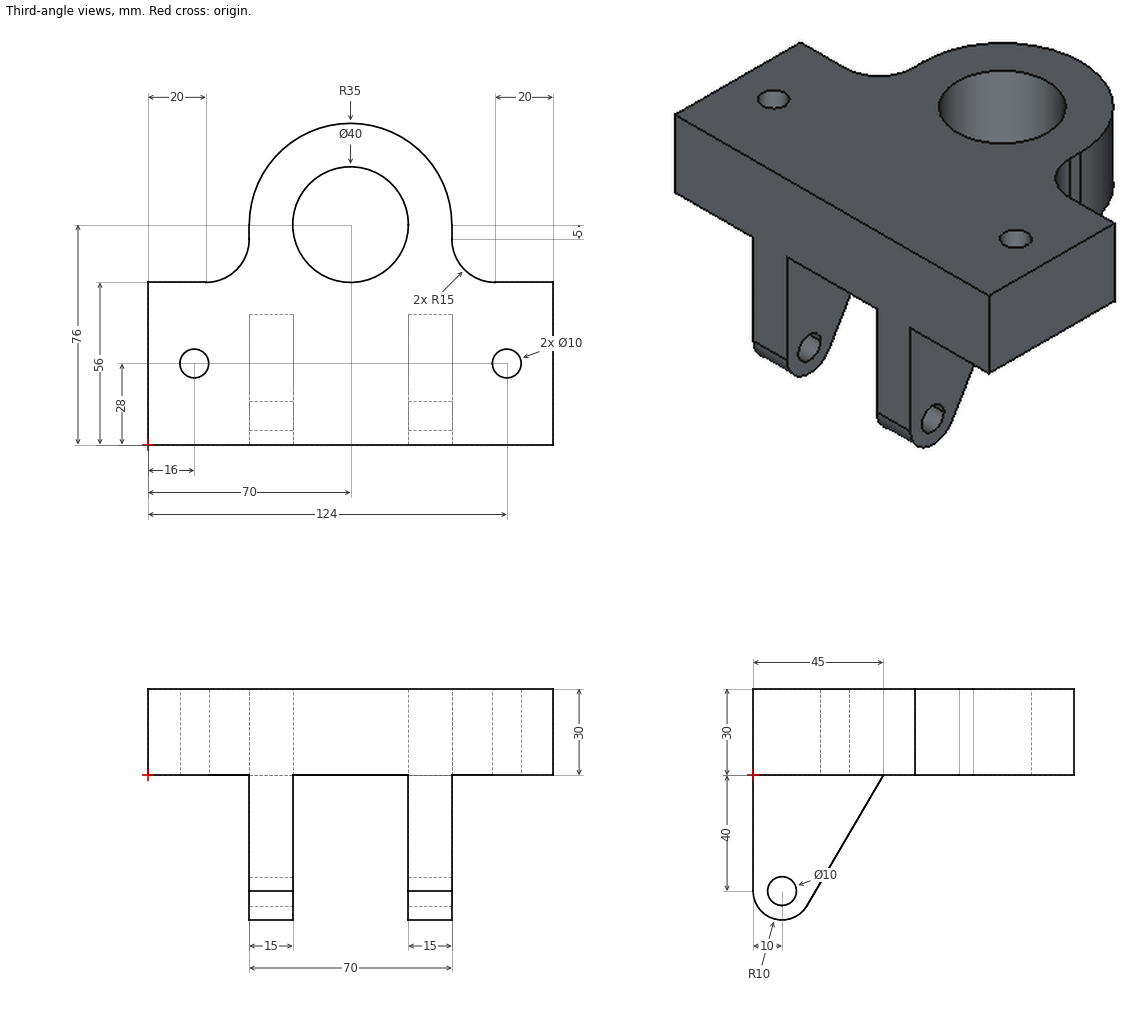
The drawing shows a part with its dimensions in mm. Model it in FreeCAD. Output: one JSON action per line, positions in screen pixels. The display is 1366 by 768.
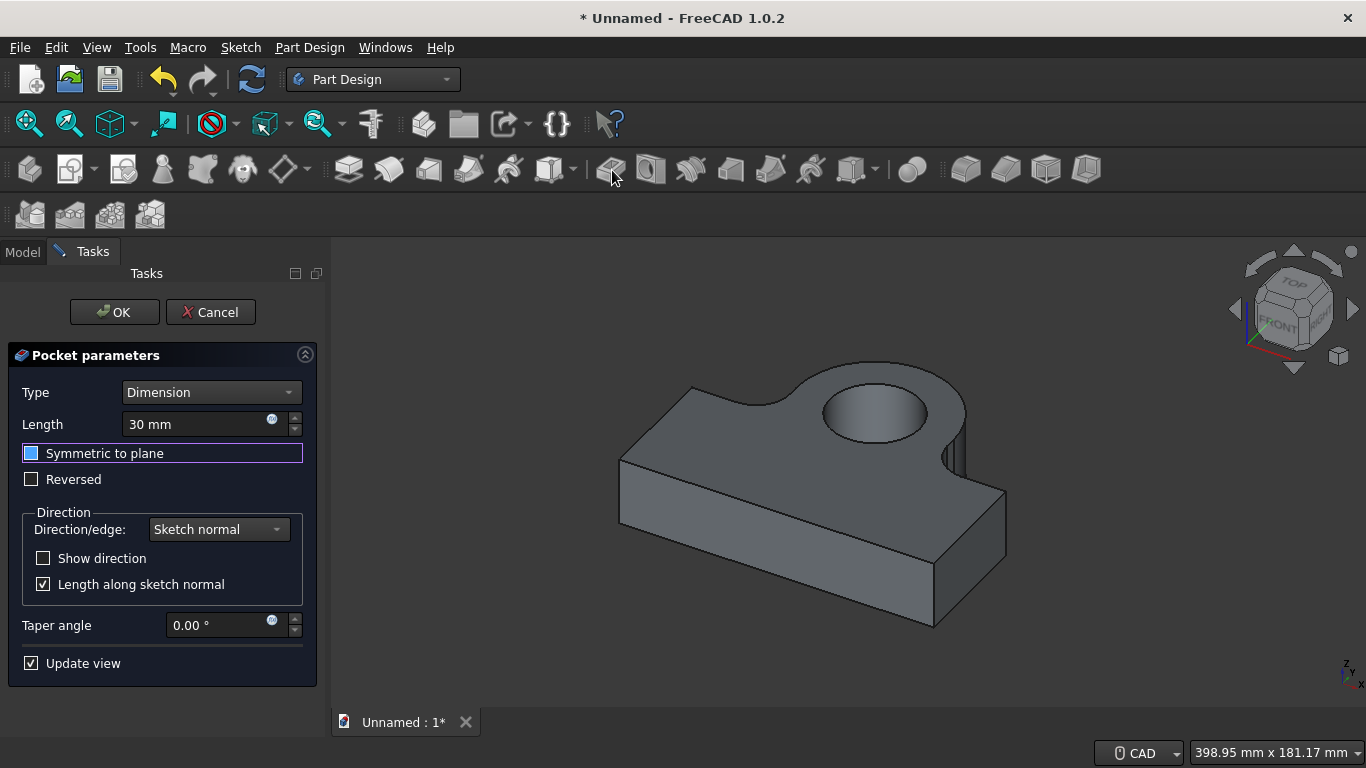
{"action": "left_click", "coordinate": [115, 312]}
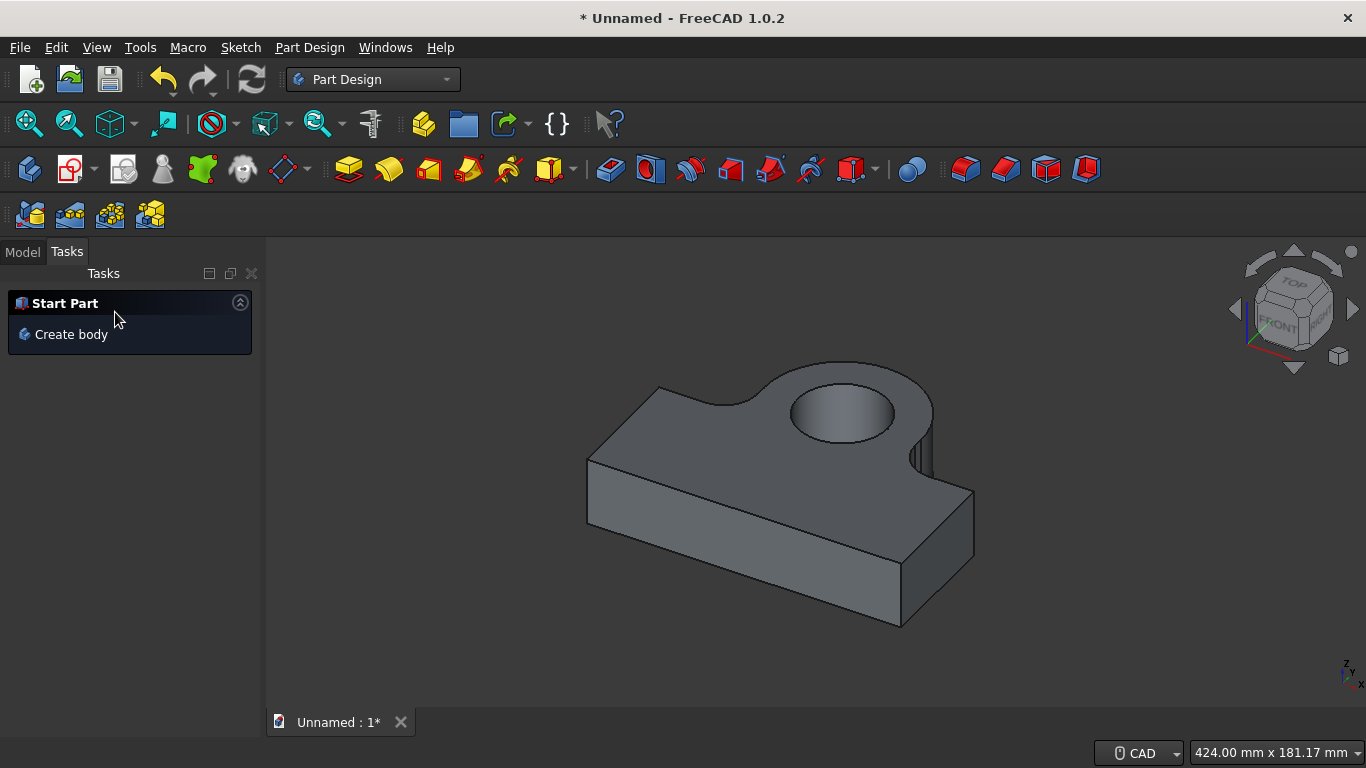
{"action": "key", "text": "6"}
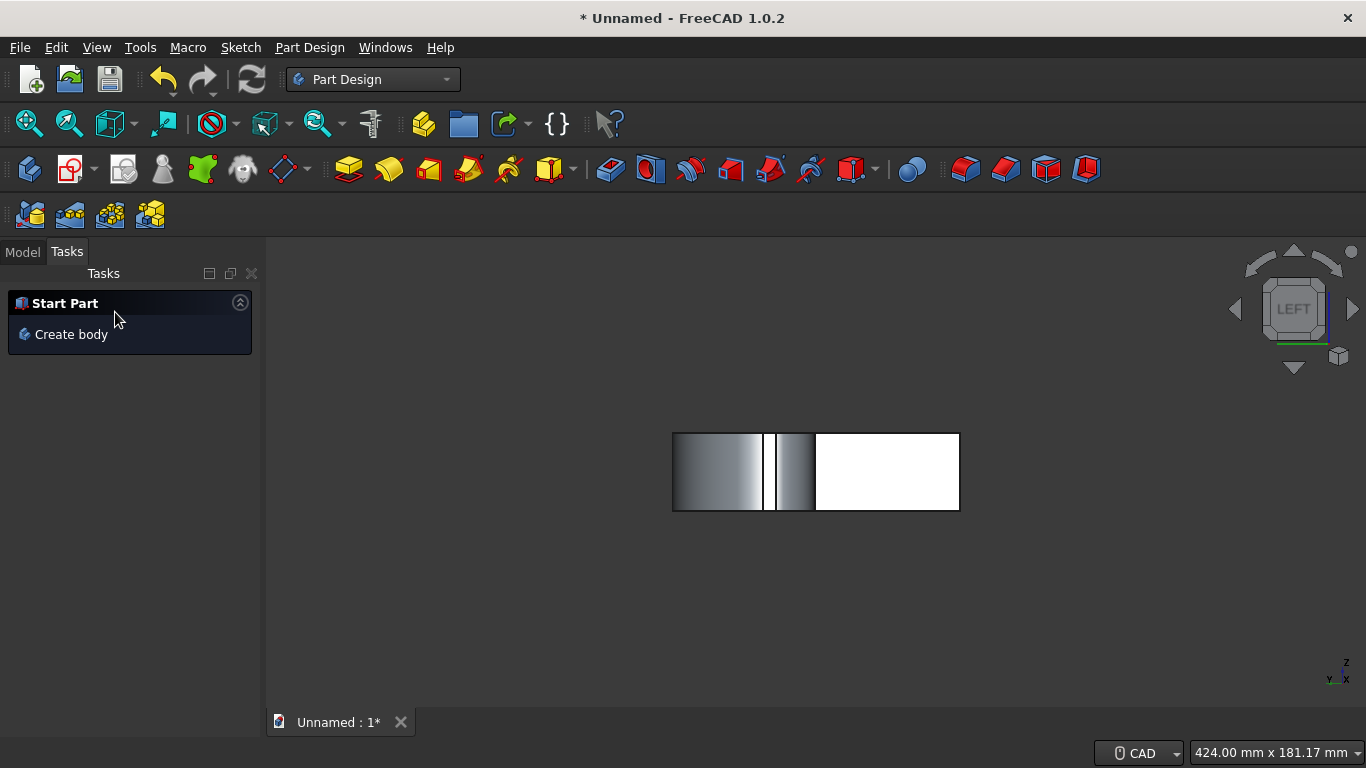
{"action": "left_click", "coordinate": [30, 124]}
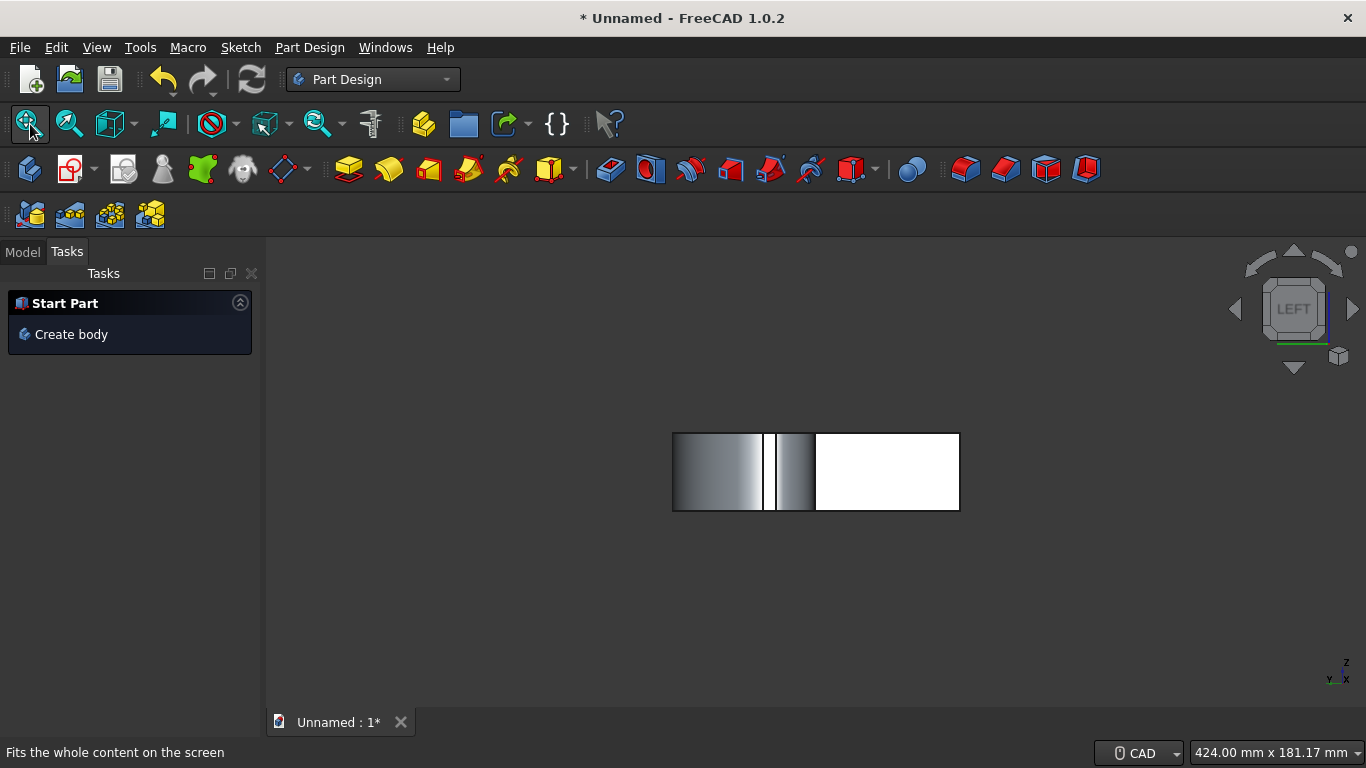
{"action": "scroll", "coordinate": [769, 449], "scroll_direction": "up", "scroll_amount": 4}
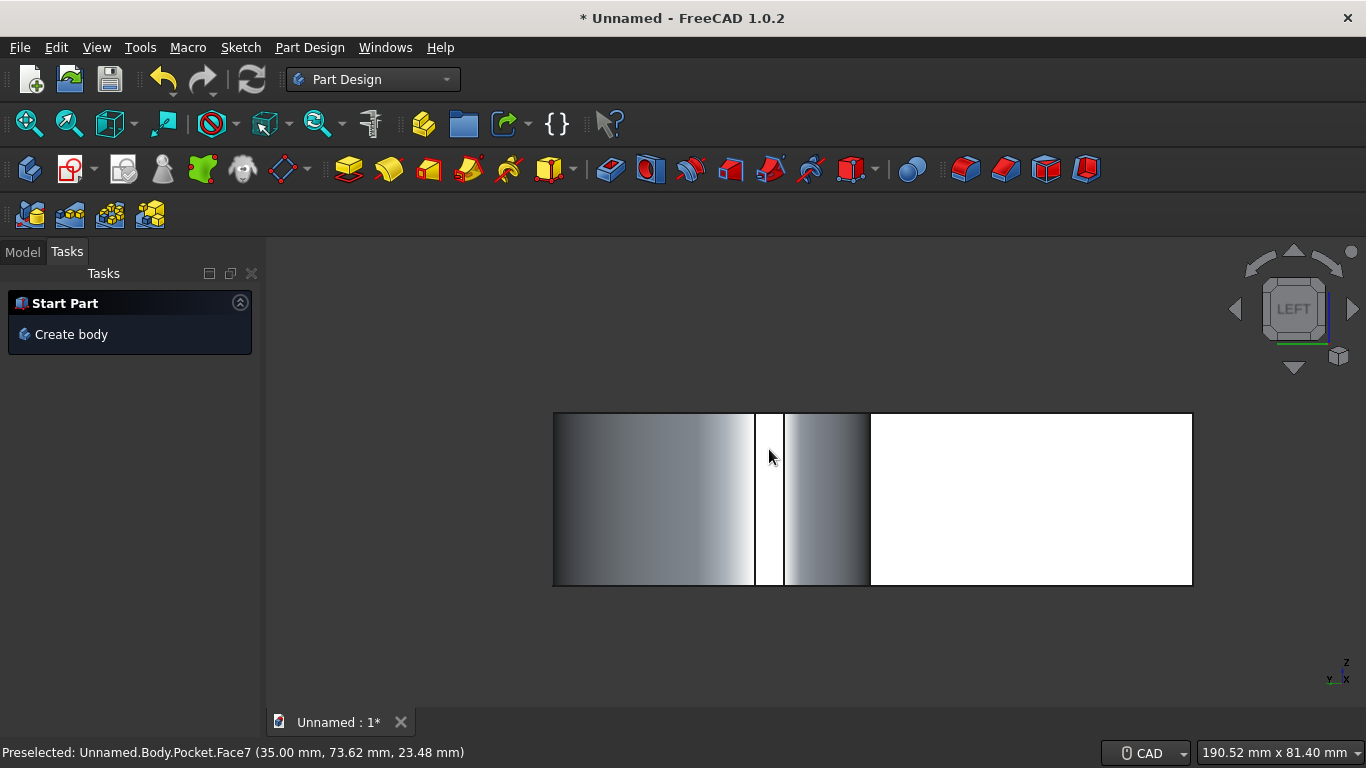
{"action": "left_click", "coordinate": [769, 449]}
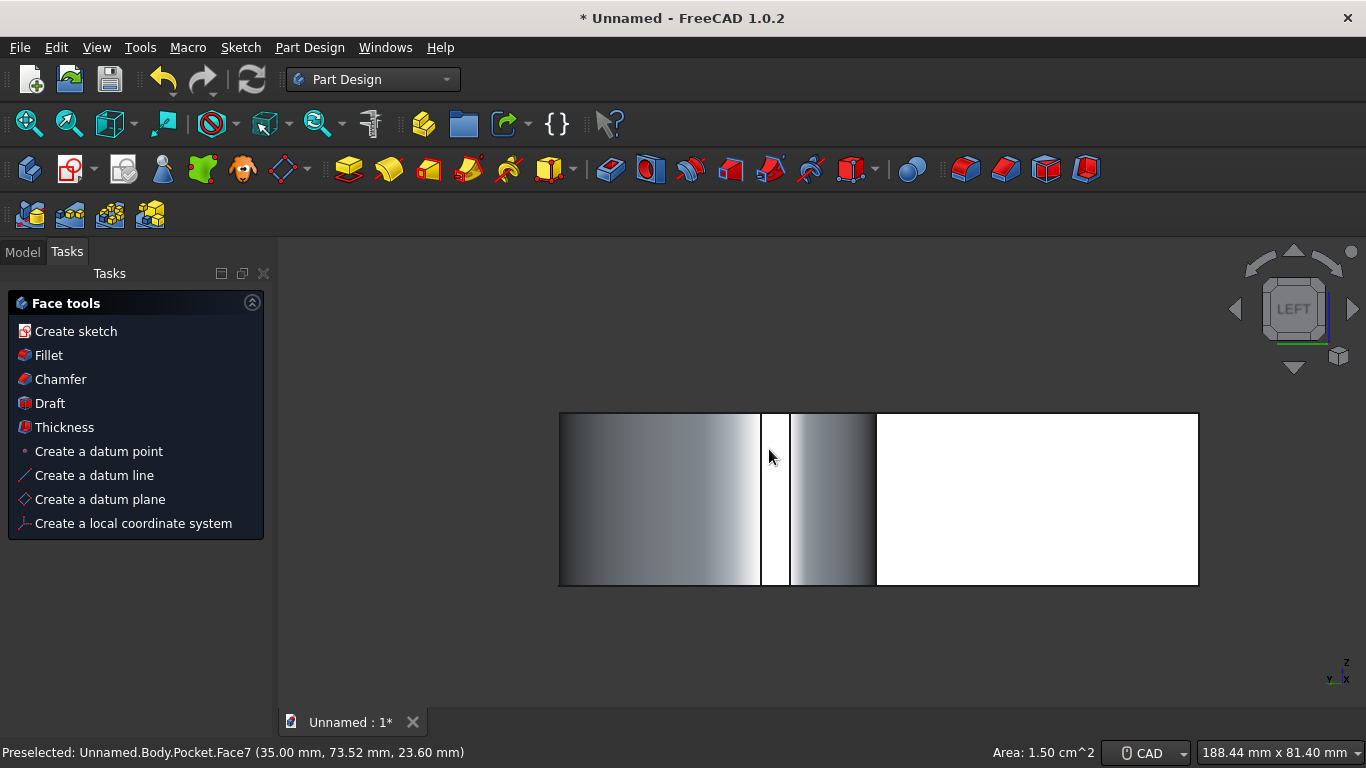
{"action": "left_click", "coordinate": [70, 170]}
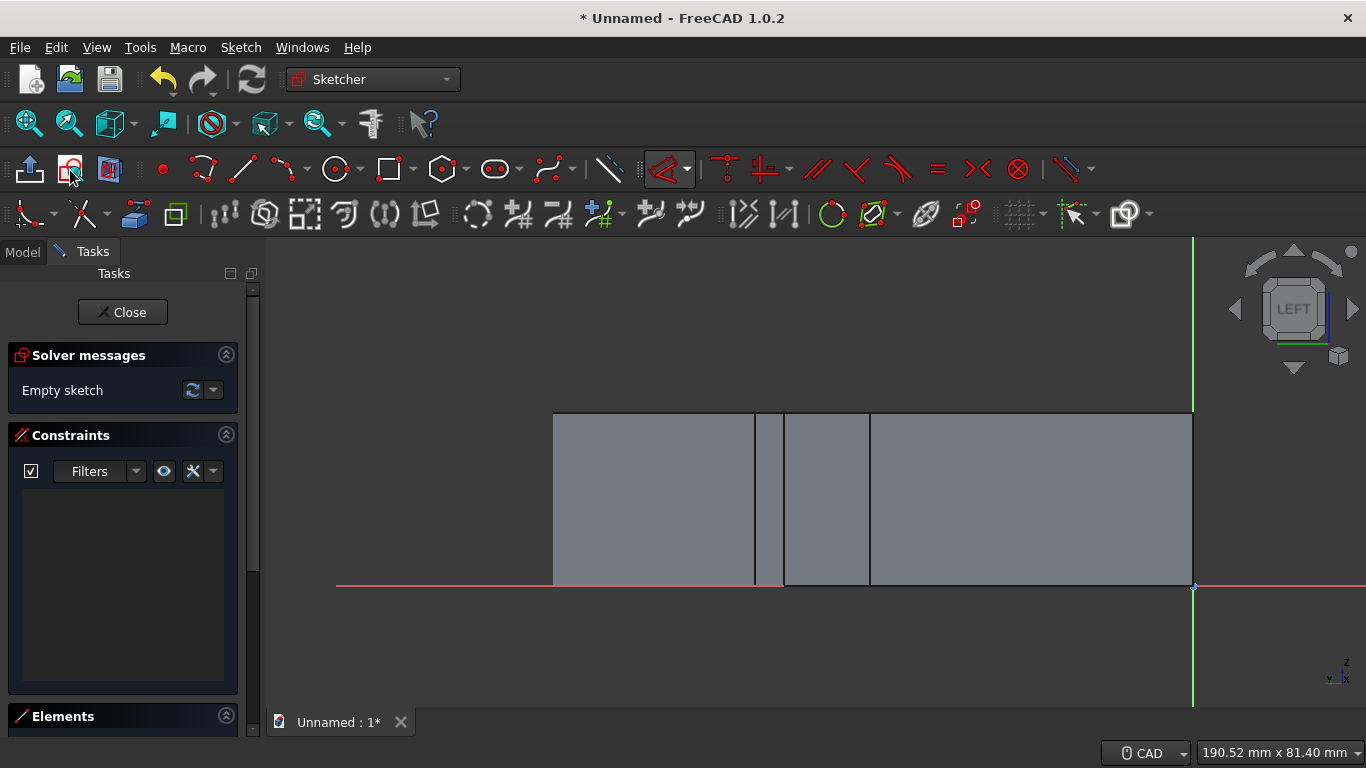
{"action": "left_click", "coordinate": [110, 170]}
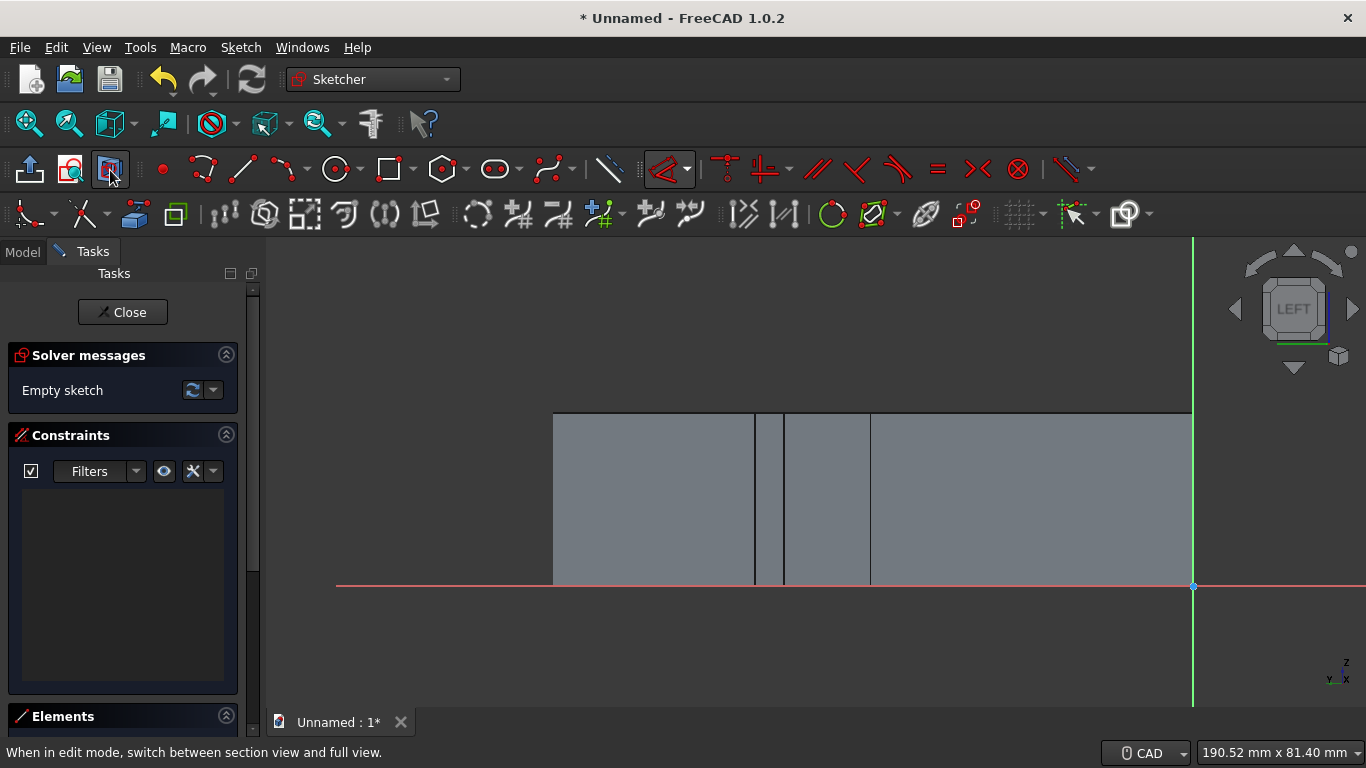
{"action": "scroll", "coordinate": [363, 265], "scroll_direction": "down", "scroll_amount": 3}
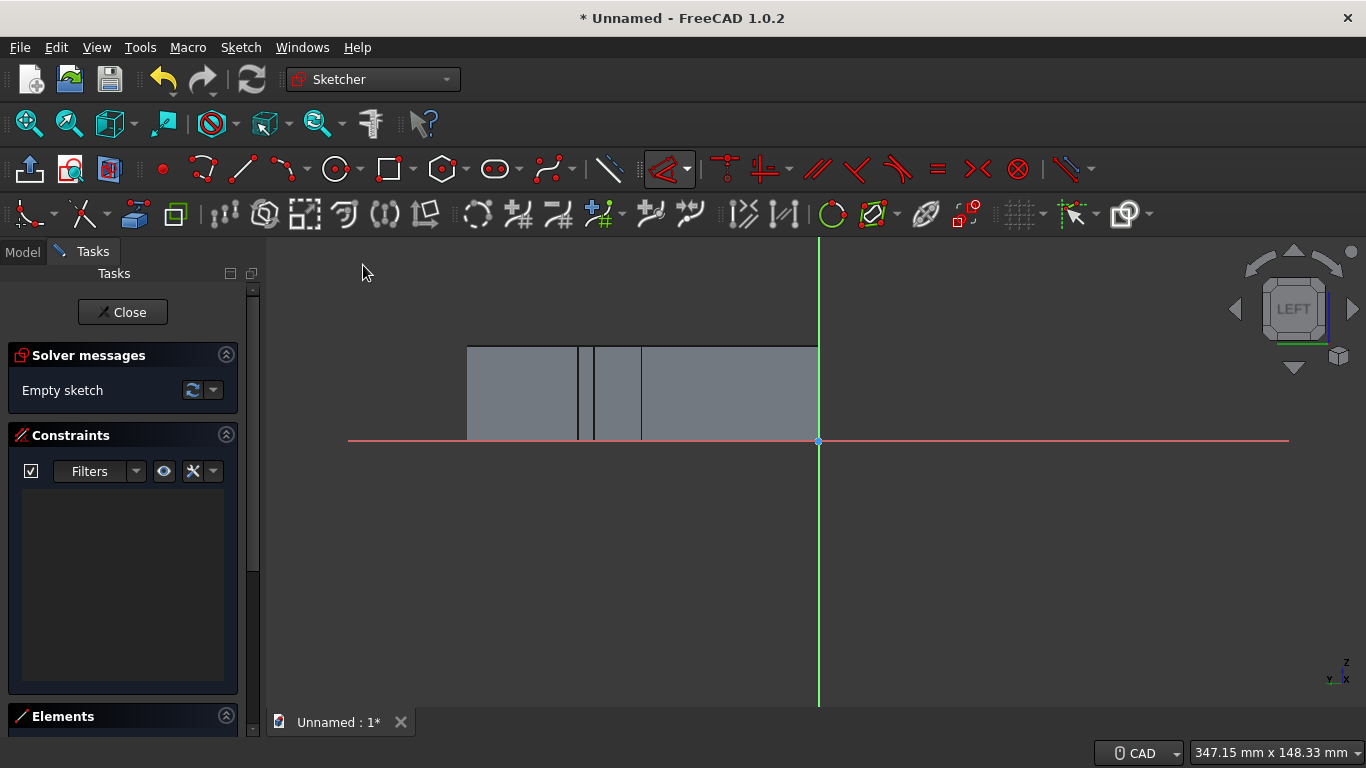
{"action": "scroll", "coordinate": [748, 578], "scroll_direction": "up", "scroll_amount": 3}